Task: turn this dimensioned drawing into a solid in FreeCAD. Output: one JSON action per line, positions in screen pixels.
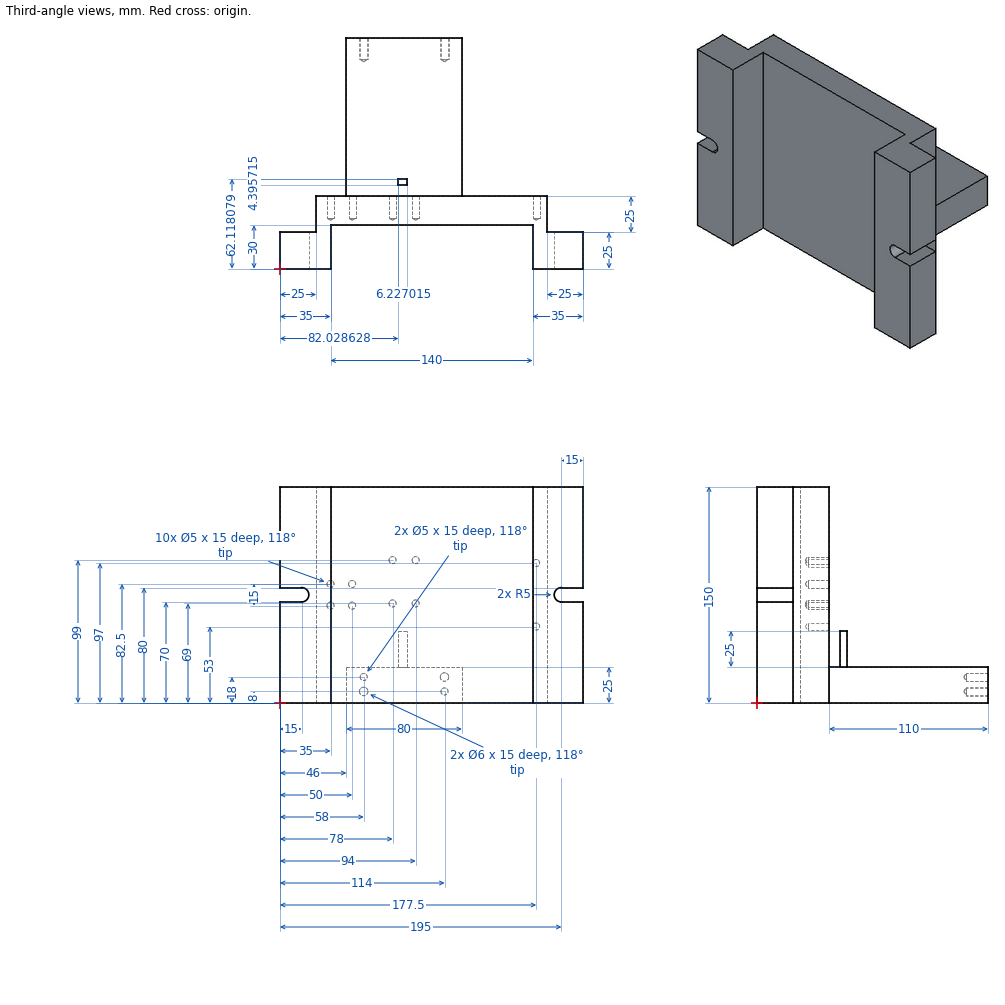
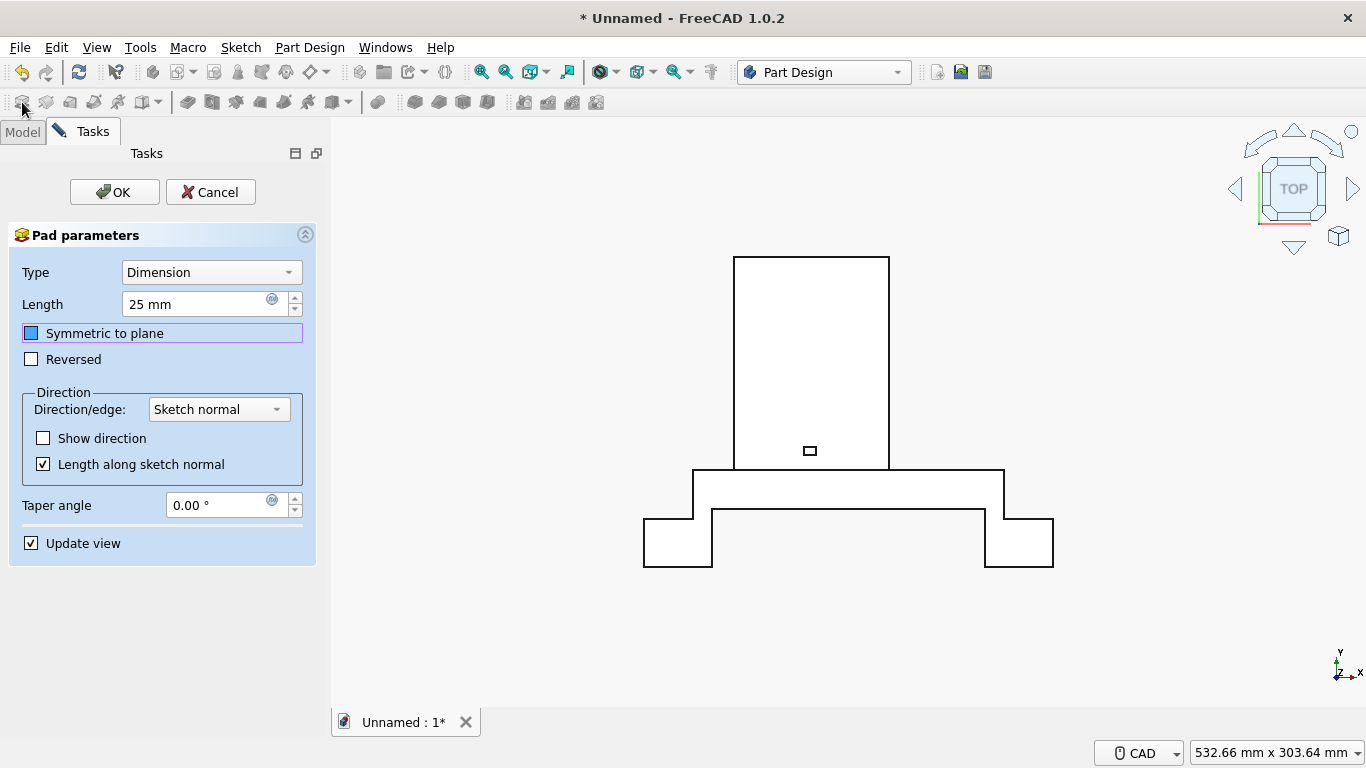
{"action": "left_click", "coordinate": [115, 192]}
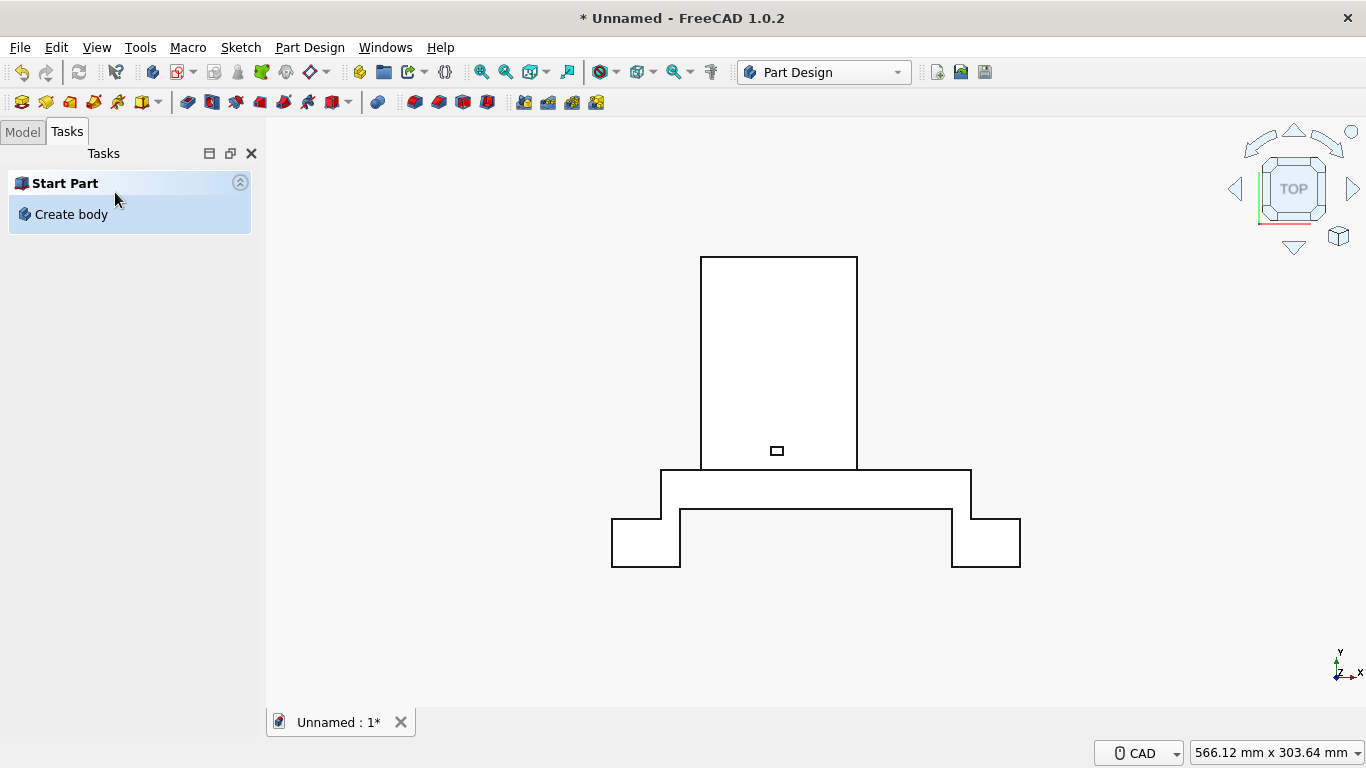
{"action": "key", "text": "0"}